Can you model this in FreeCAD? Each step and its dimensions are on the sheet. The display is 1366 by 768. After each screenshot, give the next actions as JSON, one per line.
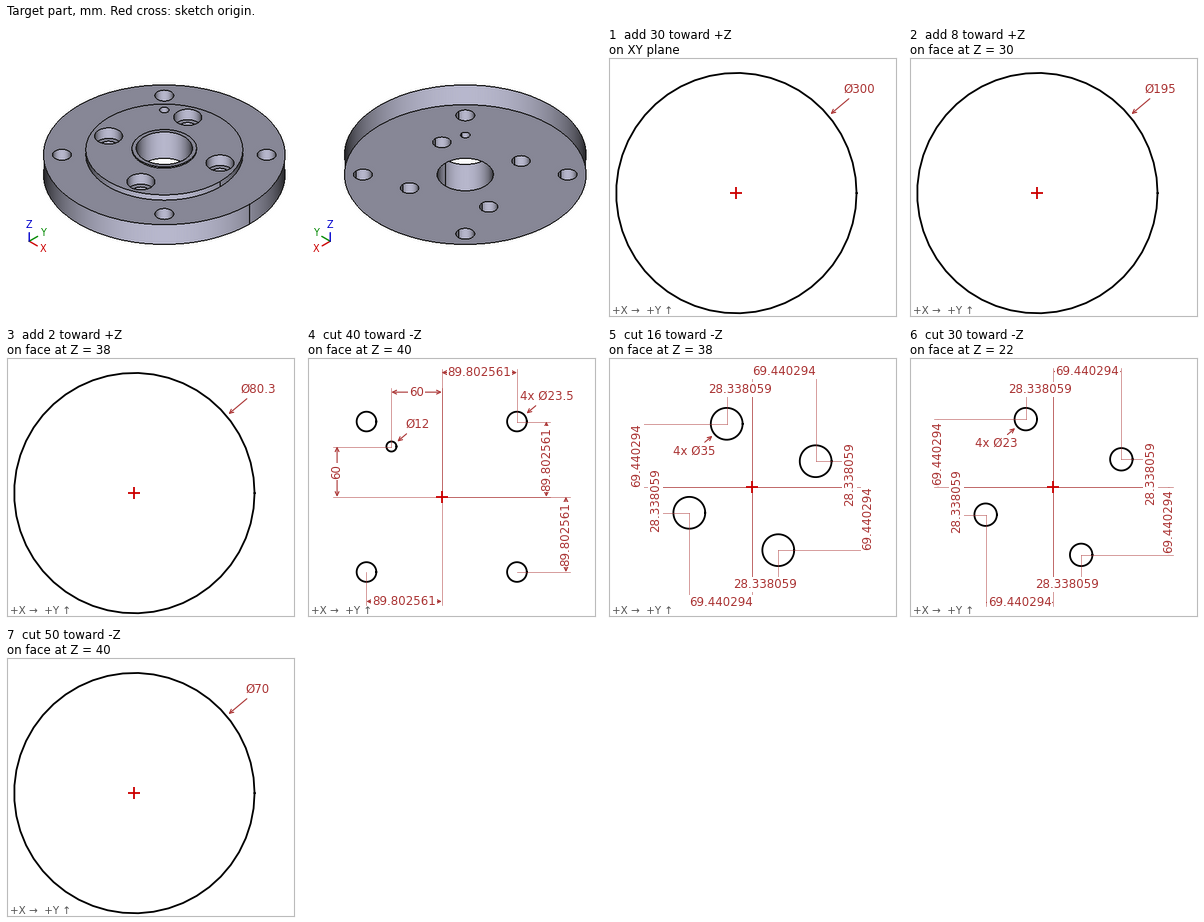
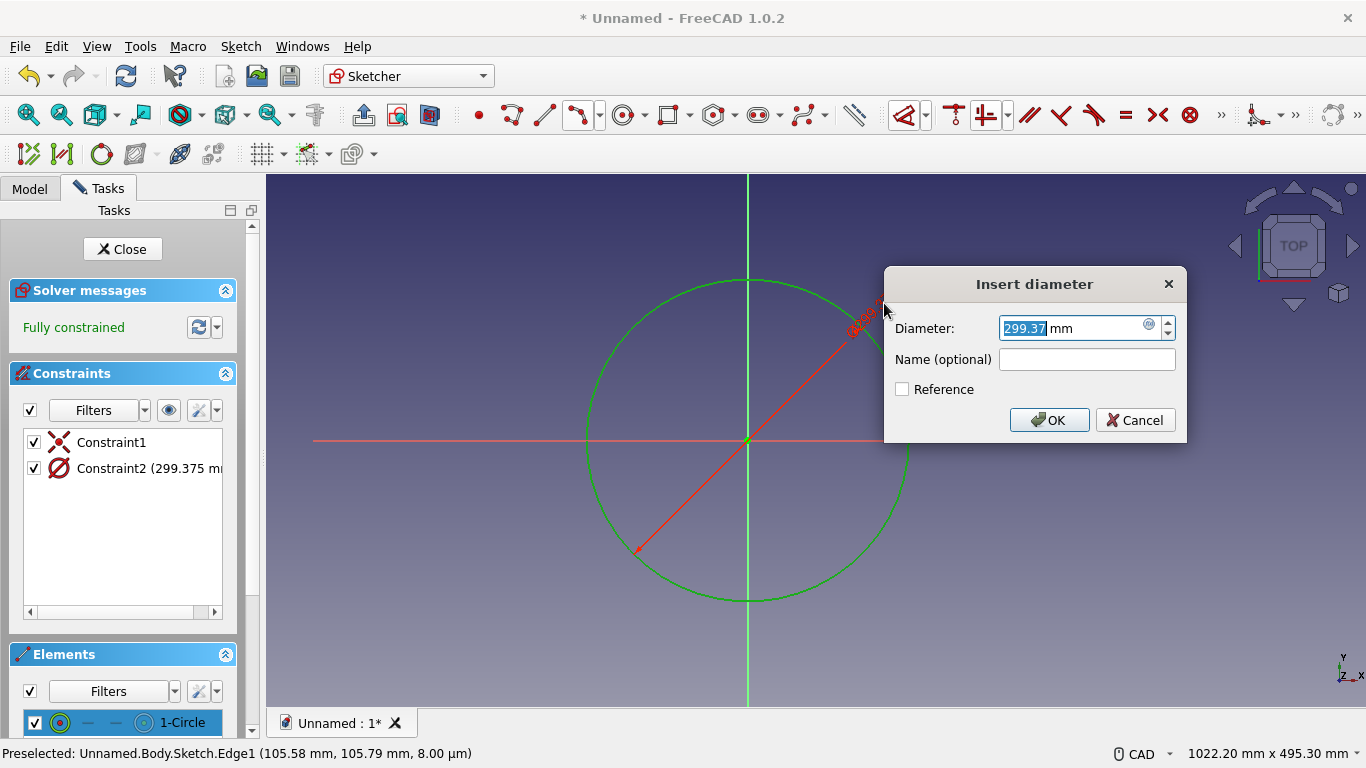
{"action": "type", "text": "300"}
{"action": "key", "text": "Return"}
{"action": "key", "text": "Escape"}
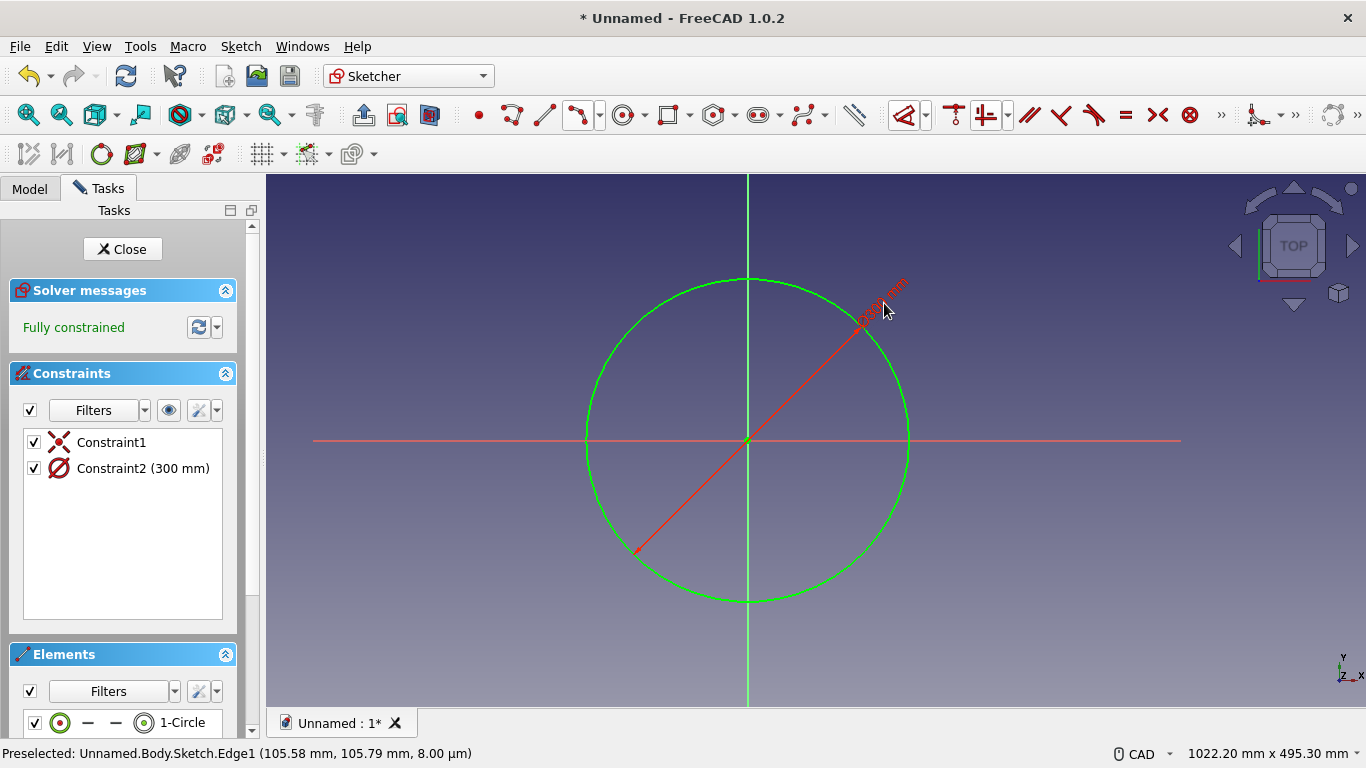
{"action": "left_click", "coordinate": [123, 249]}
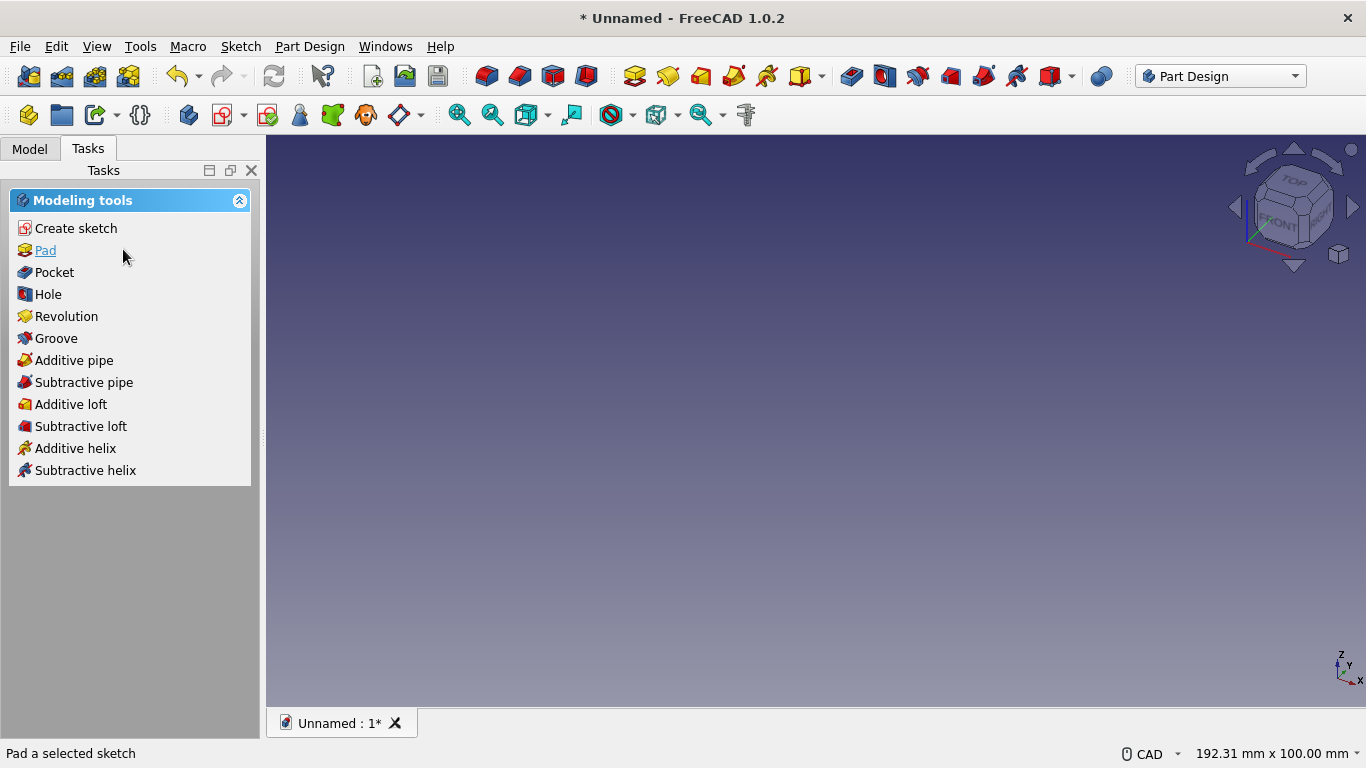
{"action": "left_click", "coordinate": [635, 76]}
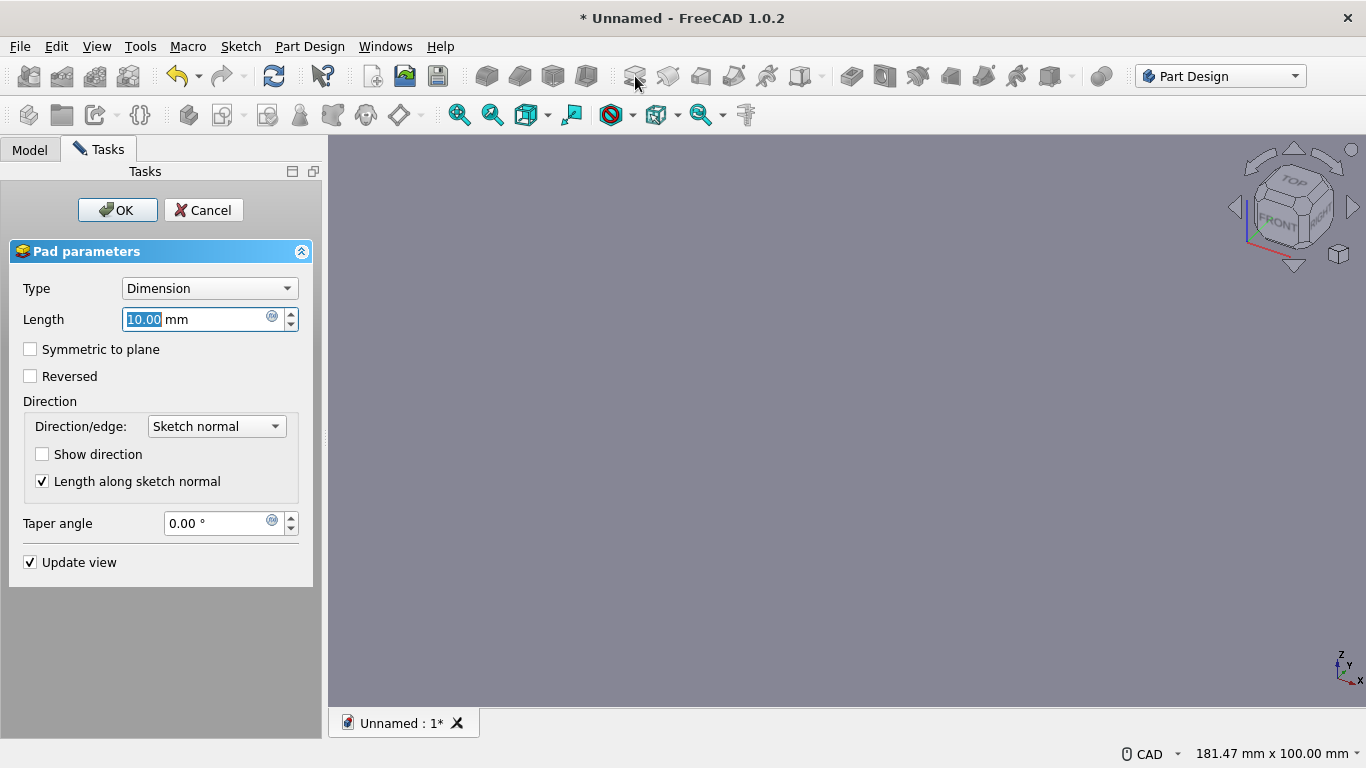
{"action": "type", "text": "30"}
{"action": "key", "text": "Tab"}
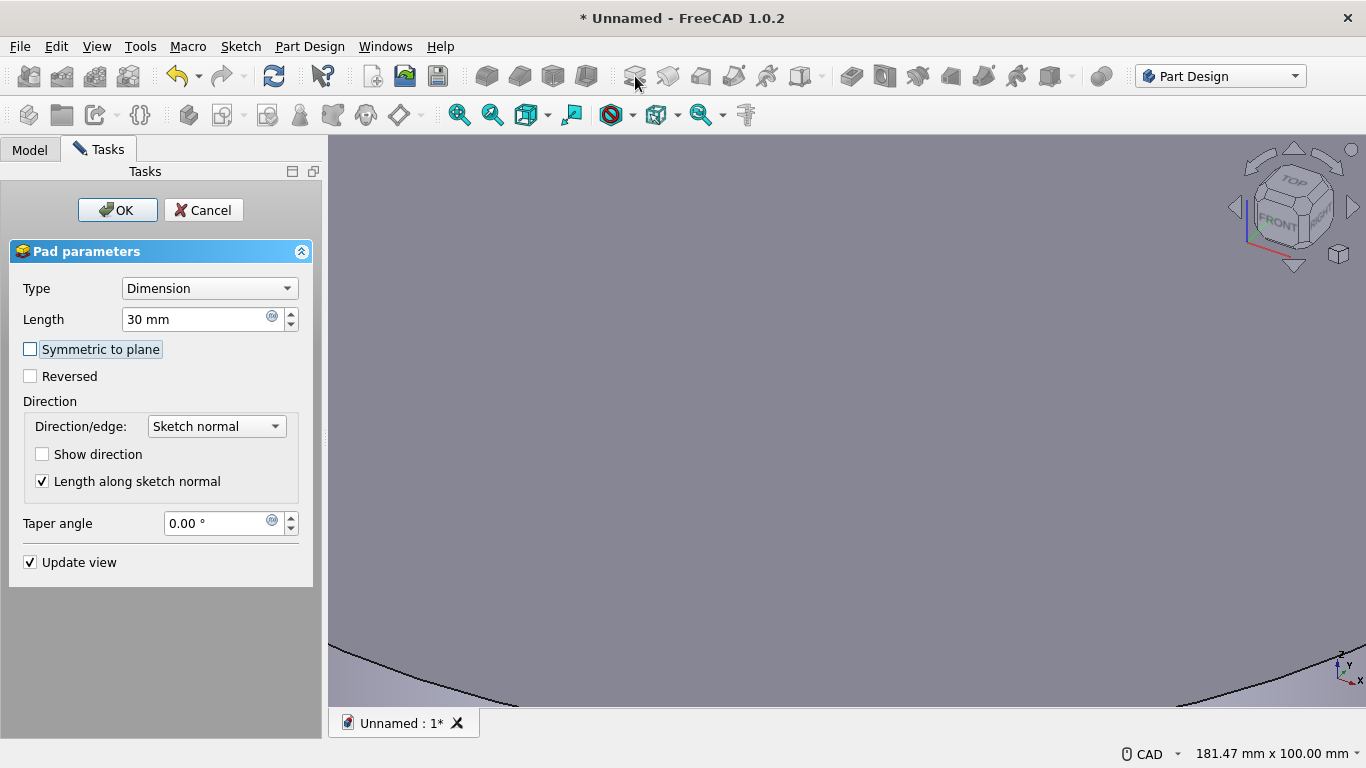
{"action": "left_click", "coordinate": [118, 210]}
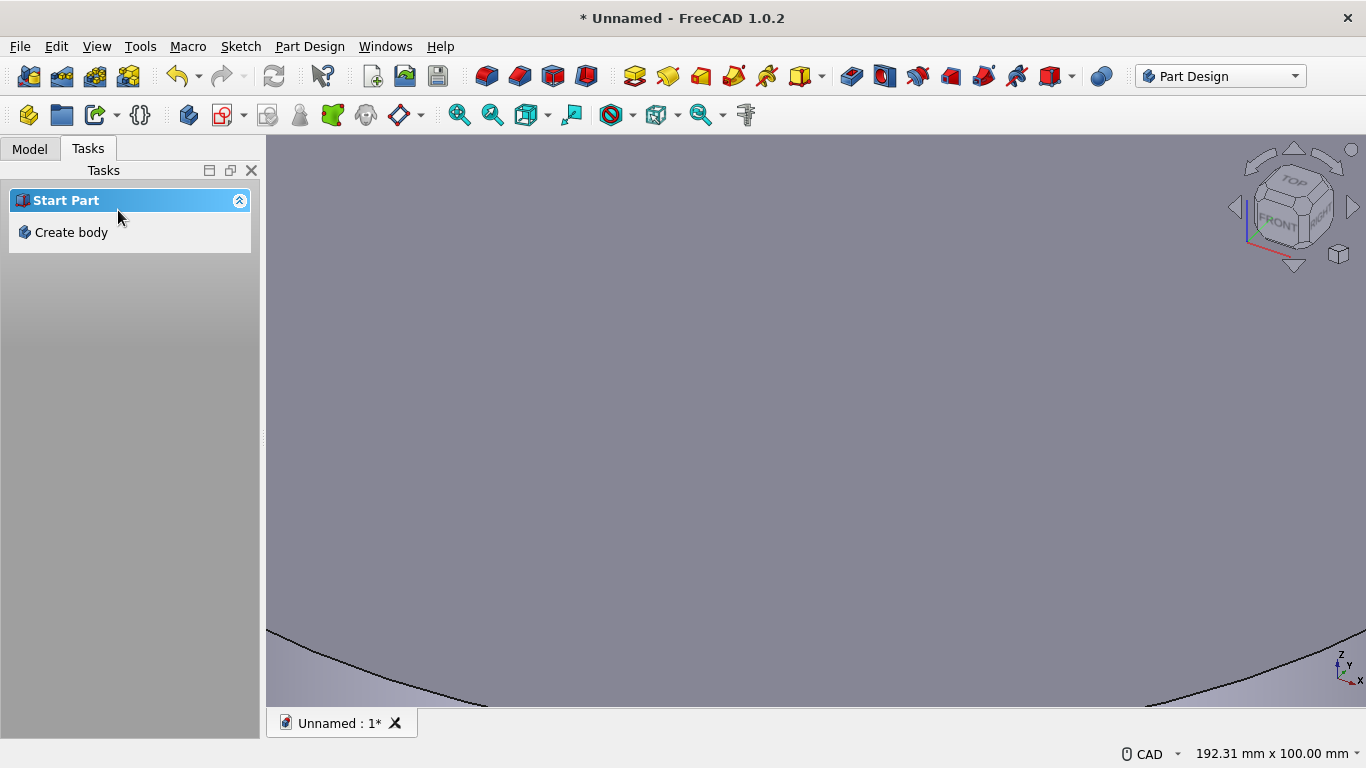
{"action": "left_click", "coordinate": [460, 116]}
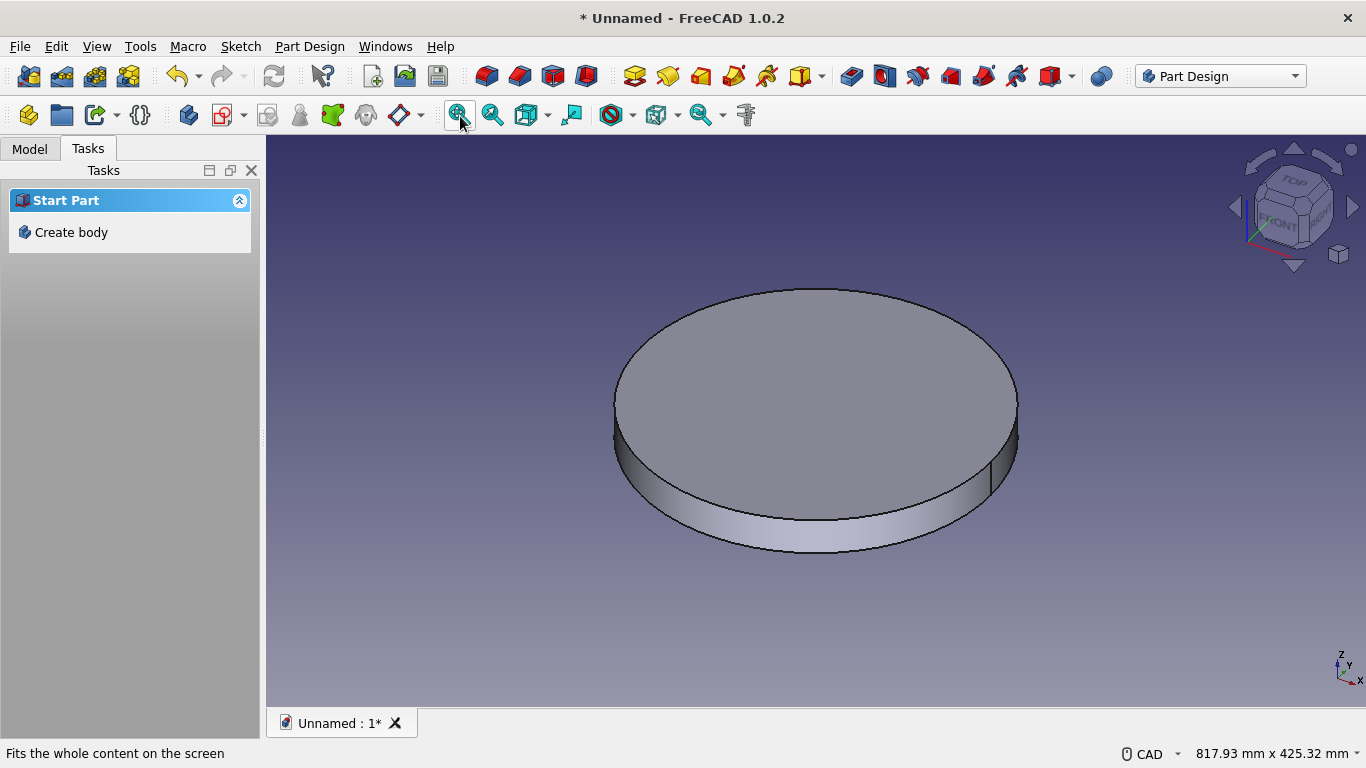
{"action": "left_click", "coordinate": [816, 403]}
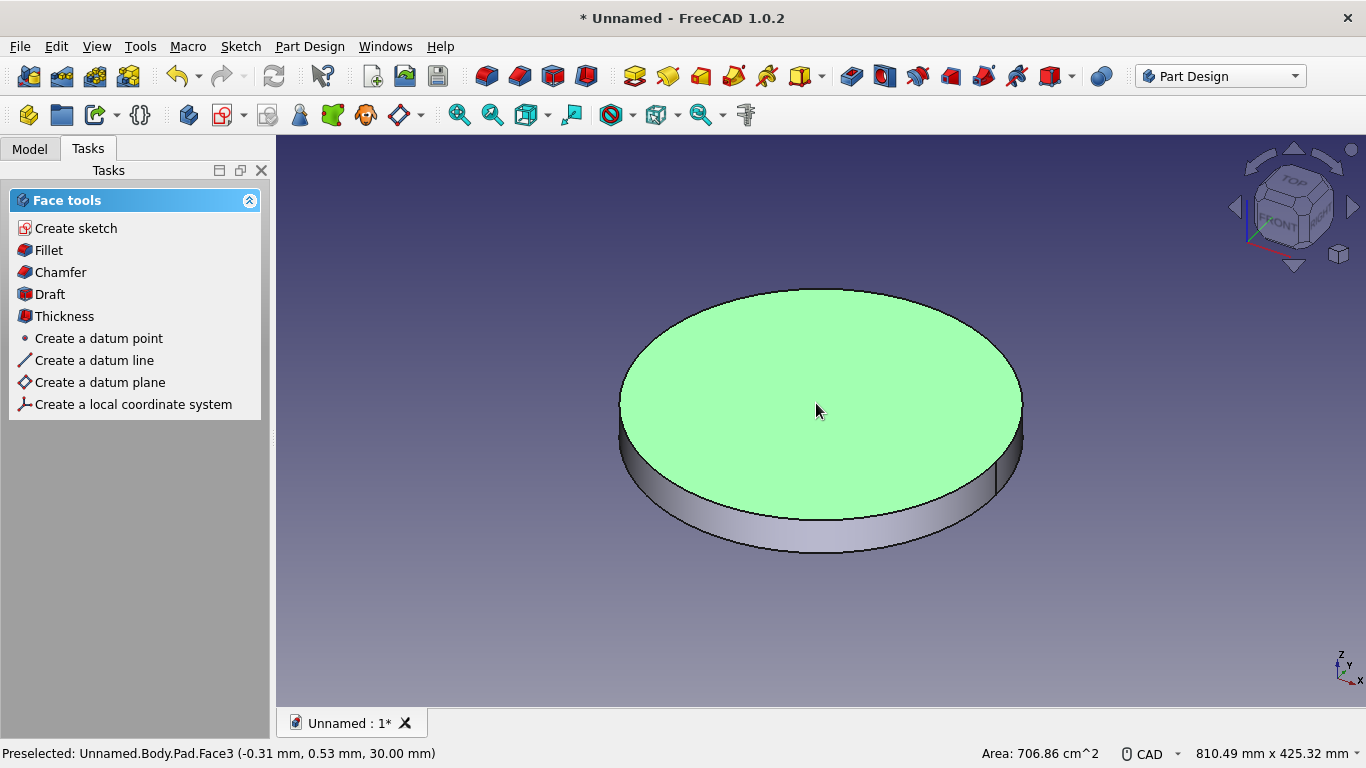
{"action": "left_click", "coordinate": [222, 116]}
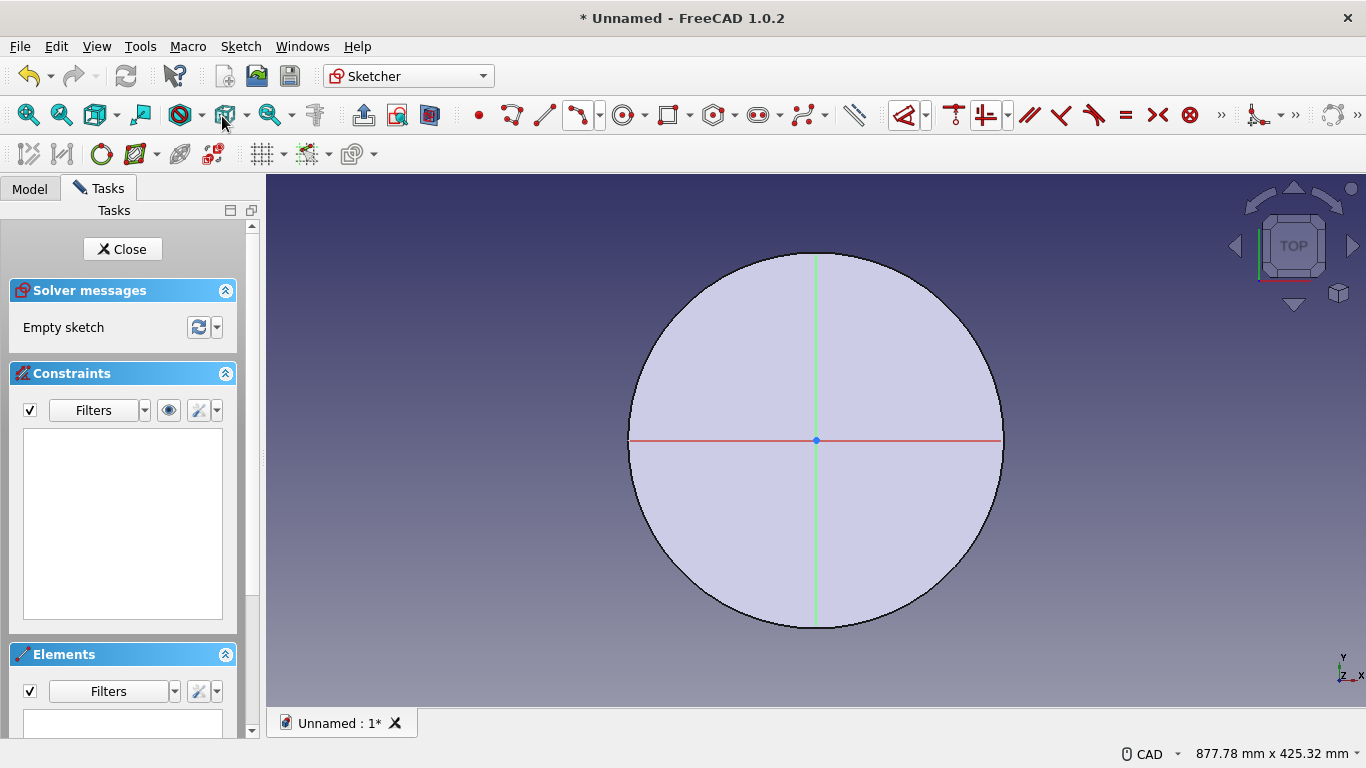
{"action": "scroll", "coordinate": [955, 440], "scroll_direction": "up", "scroll_amount": 2}